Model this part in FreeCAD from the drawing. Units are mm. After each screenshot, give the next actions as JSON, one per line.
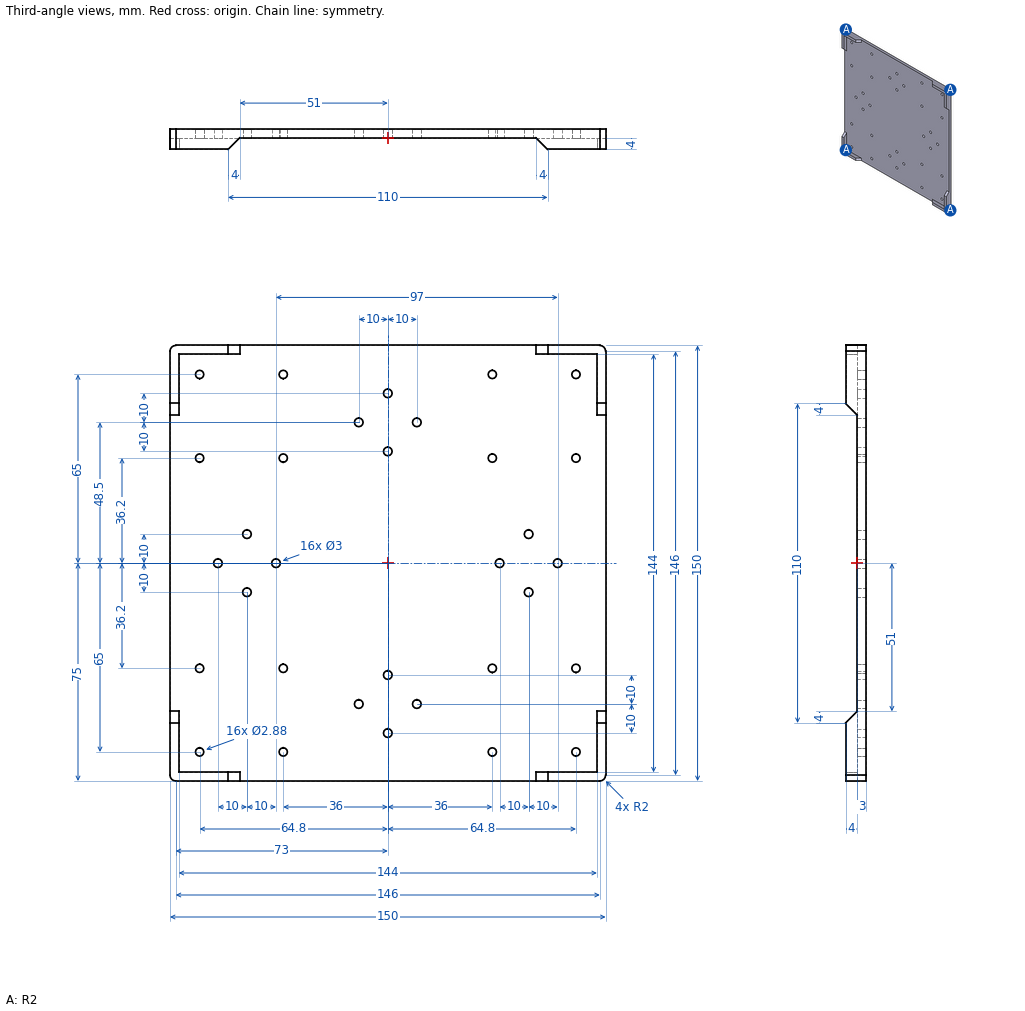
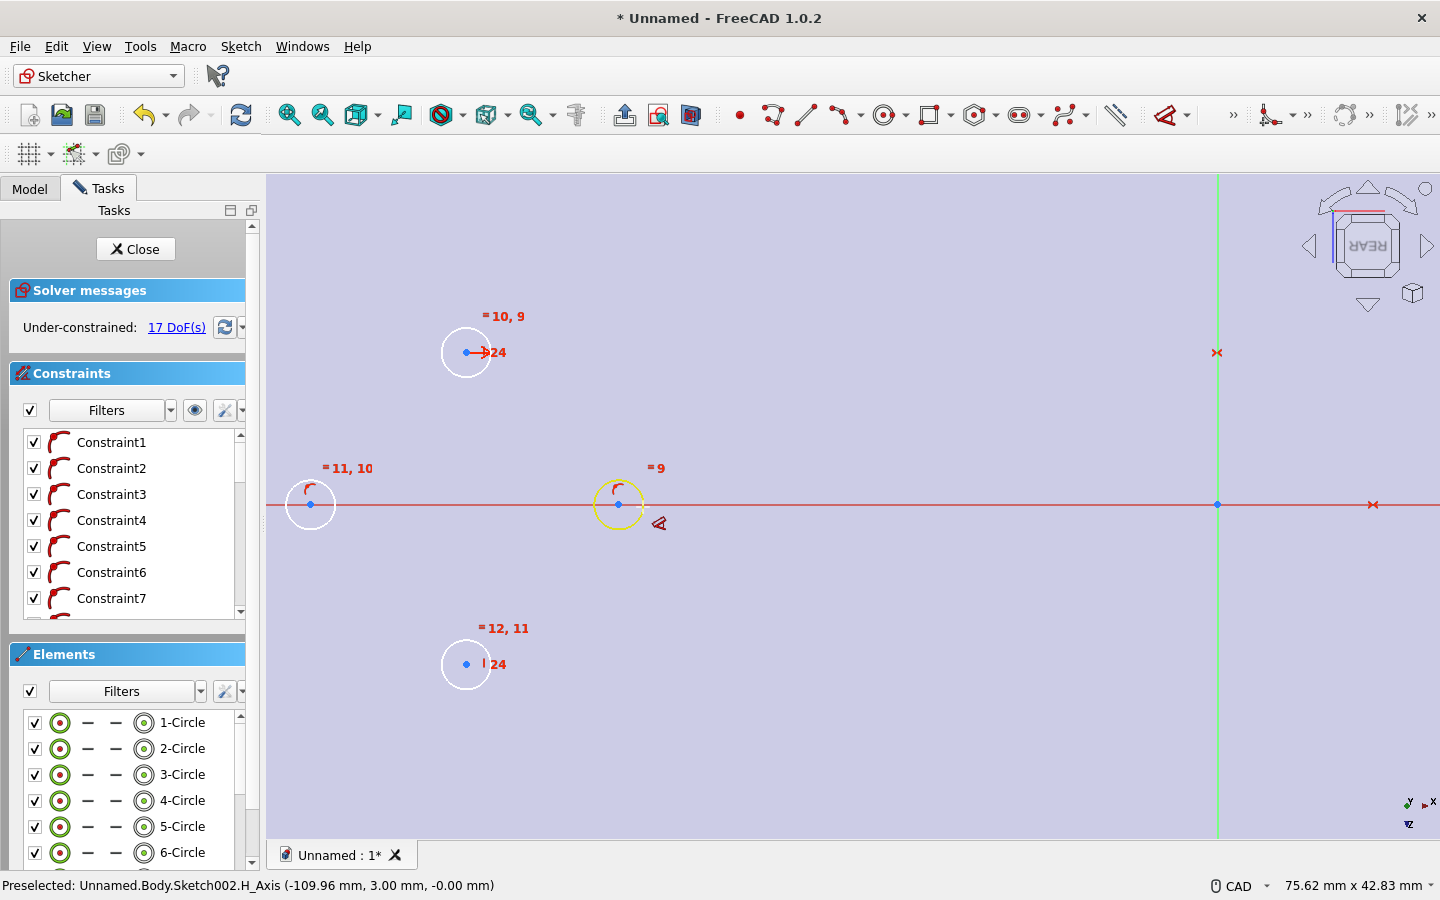
{"action": "left_click", "coordinate": [643, 506]}
{"action": "left_click", "coordinate": [667, 534]}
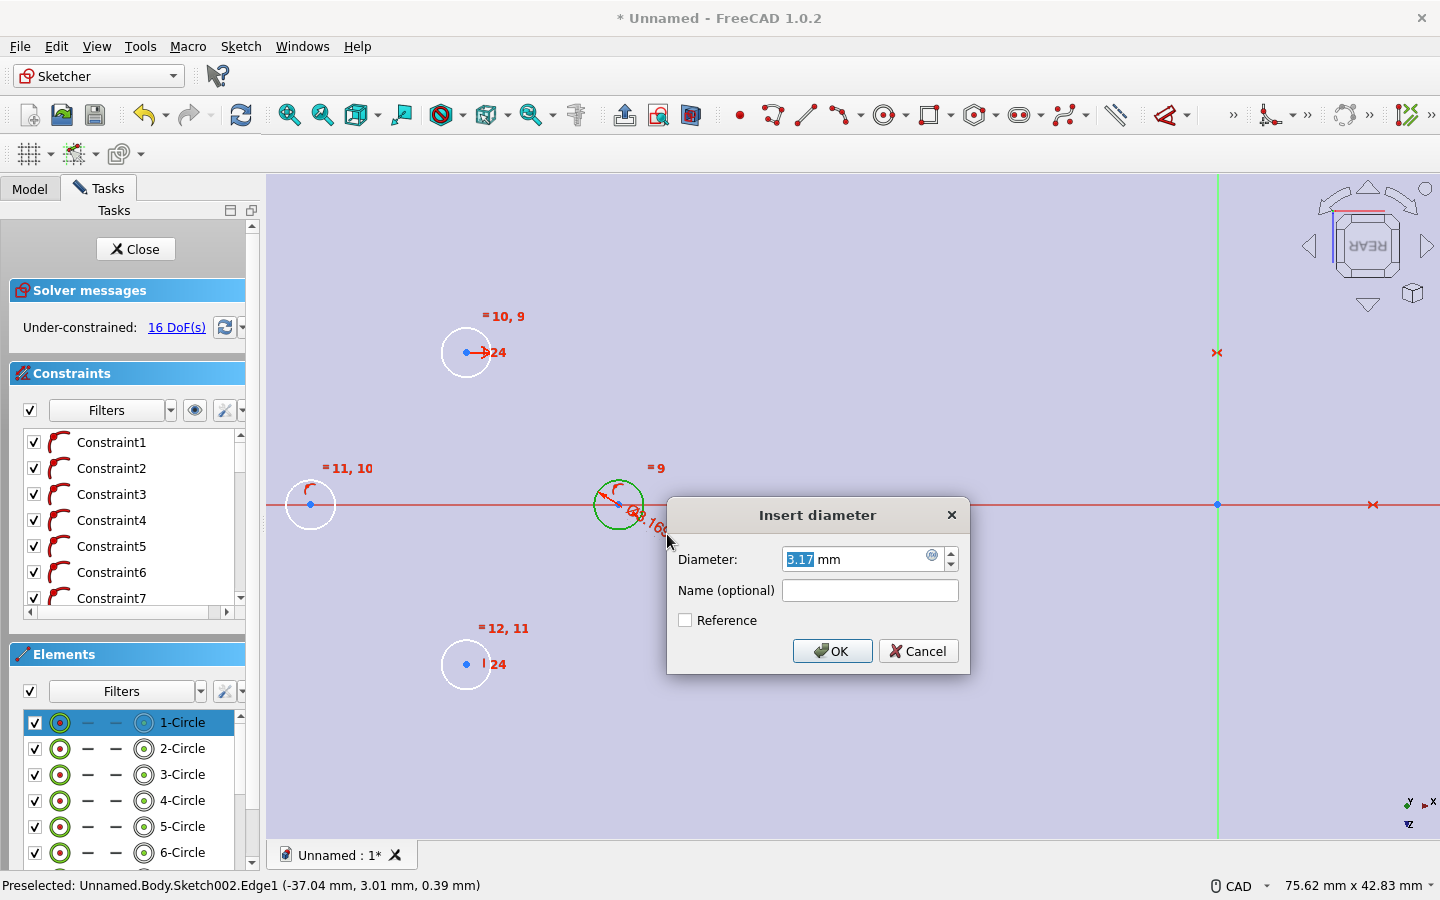
{"action": "type", "text": "3"}
{"action": "key", "text": "Return"}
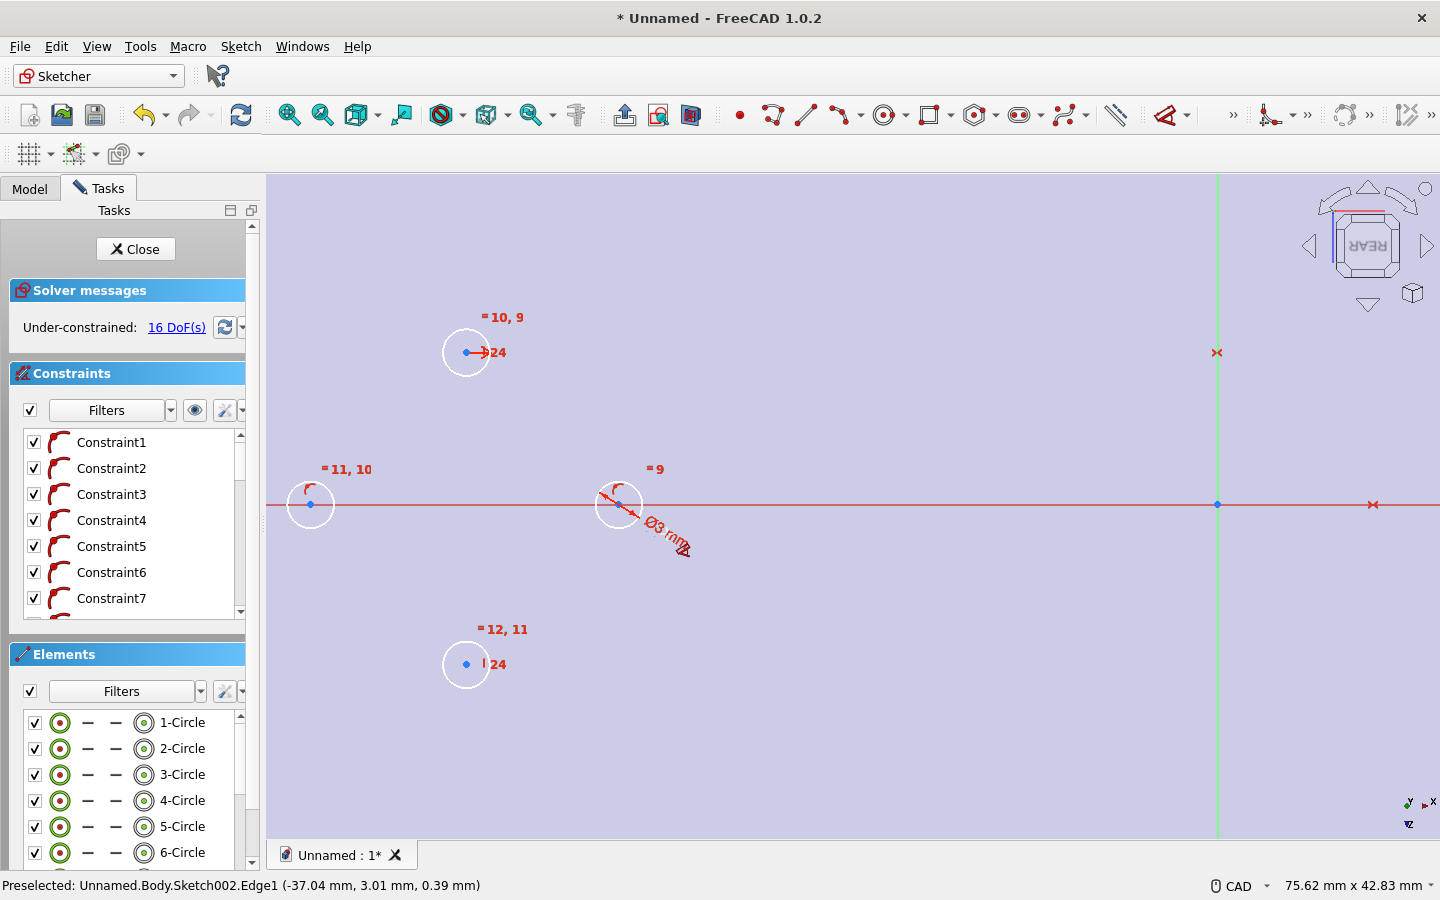
{"action": "scroll", "coordinate": [643, 507], "scroll_direction": "down", "scroll_amount": 7}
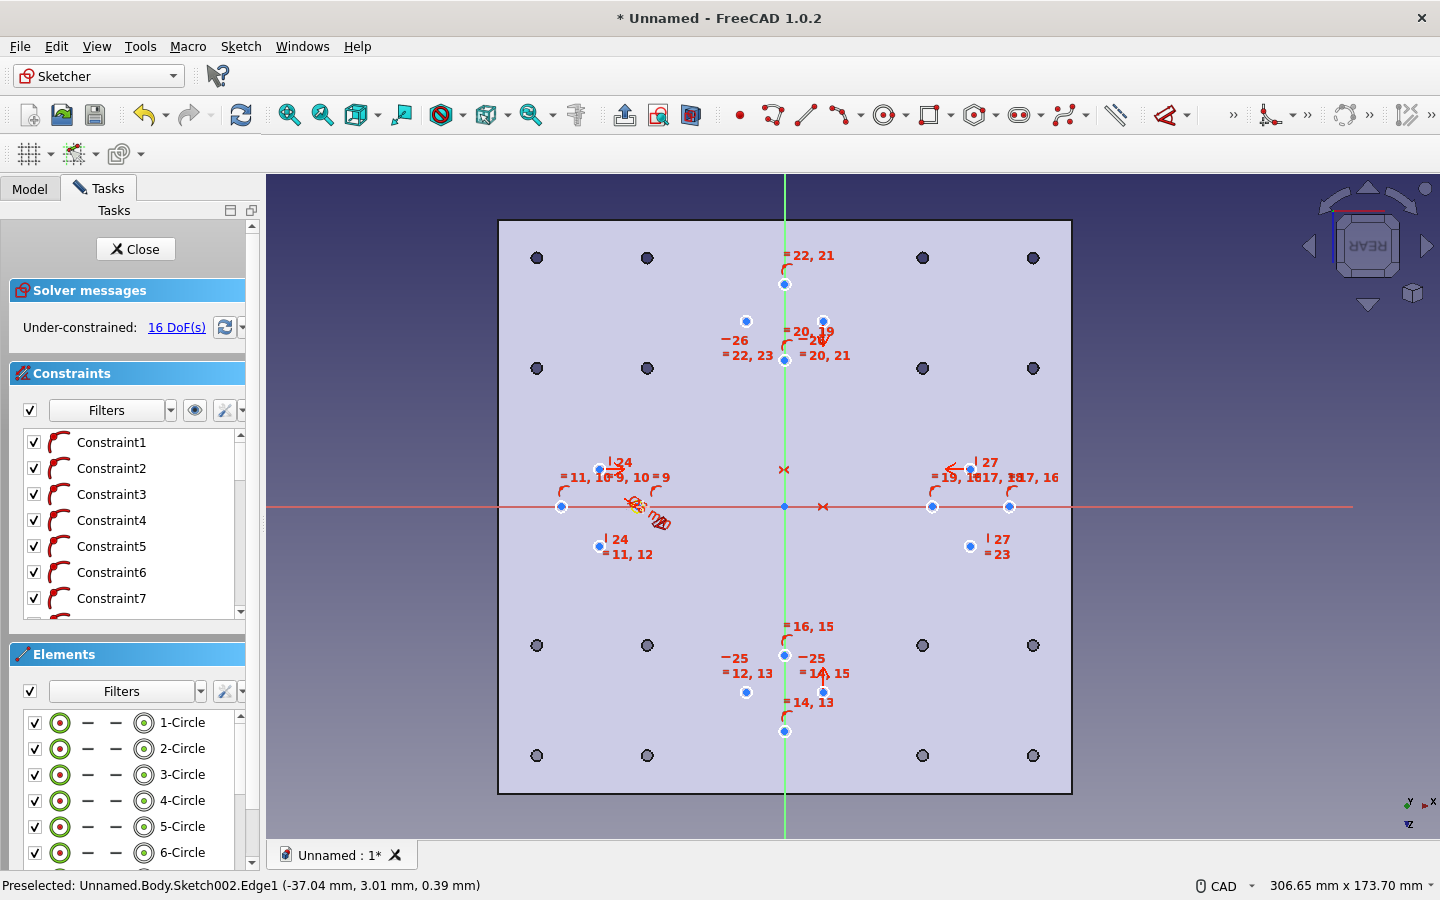
{"action": "left_click", "coordinate": [600, 469]}
{"action": "left_click", "coordinate": [566, 488]}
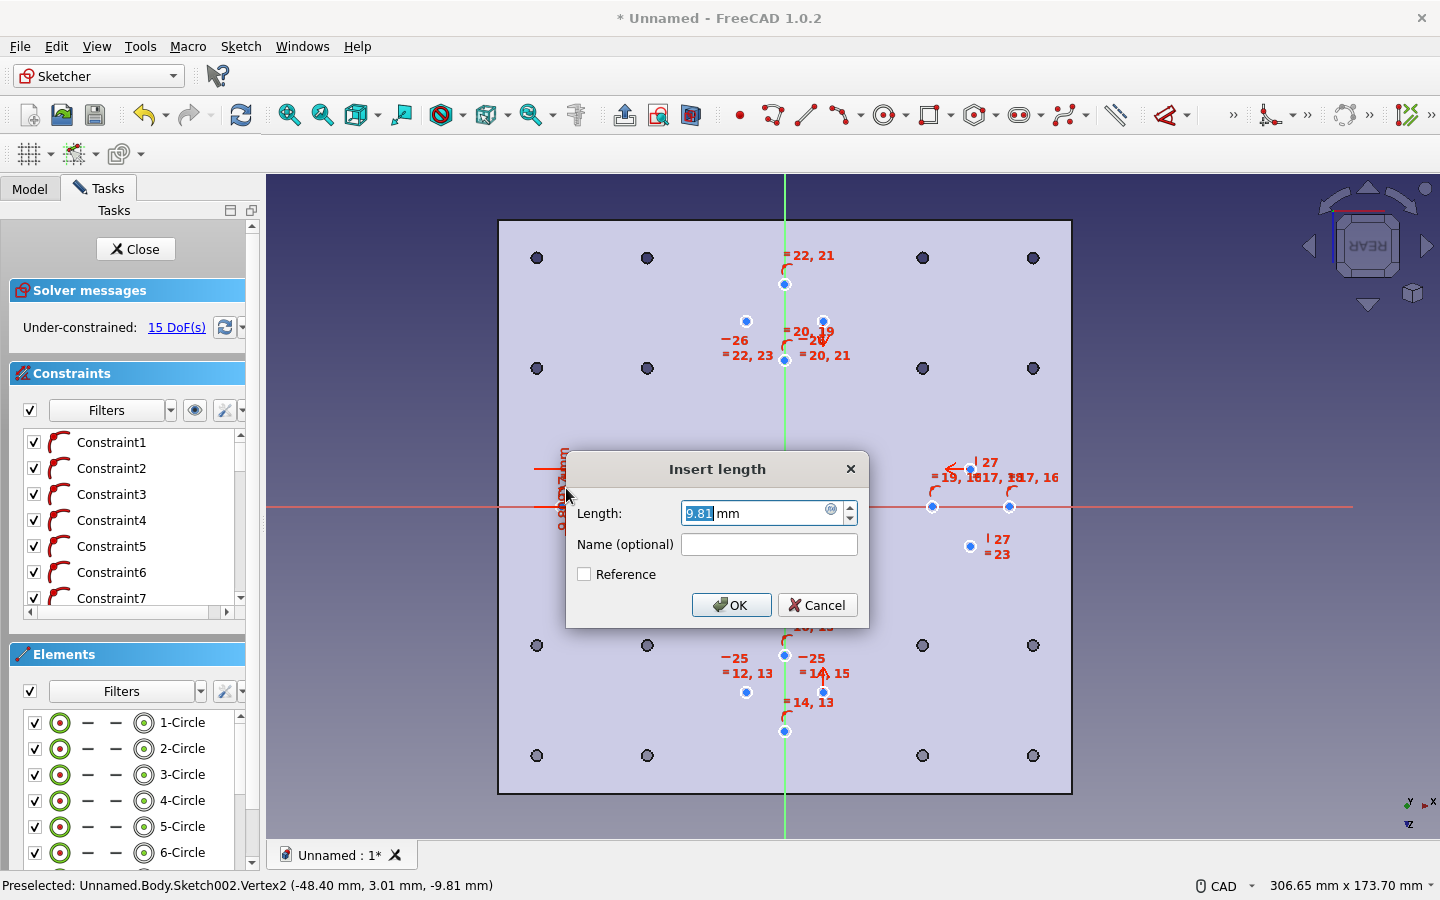
{"action": "type", "text": "10"}
{"action": "key", "text": "Return"}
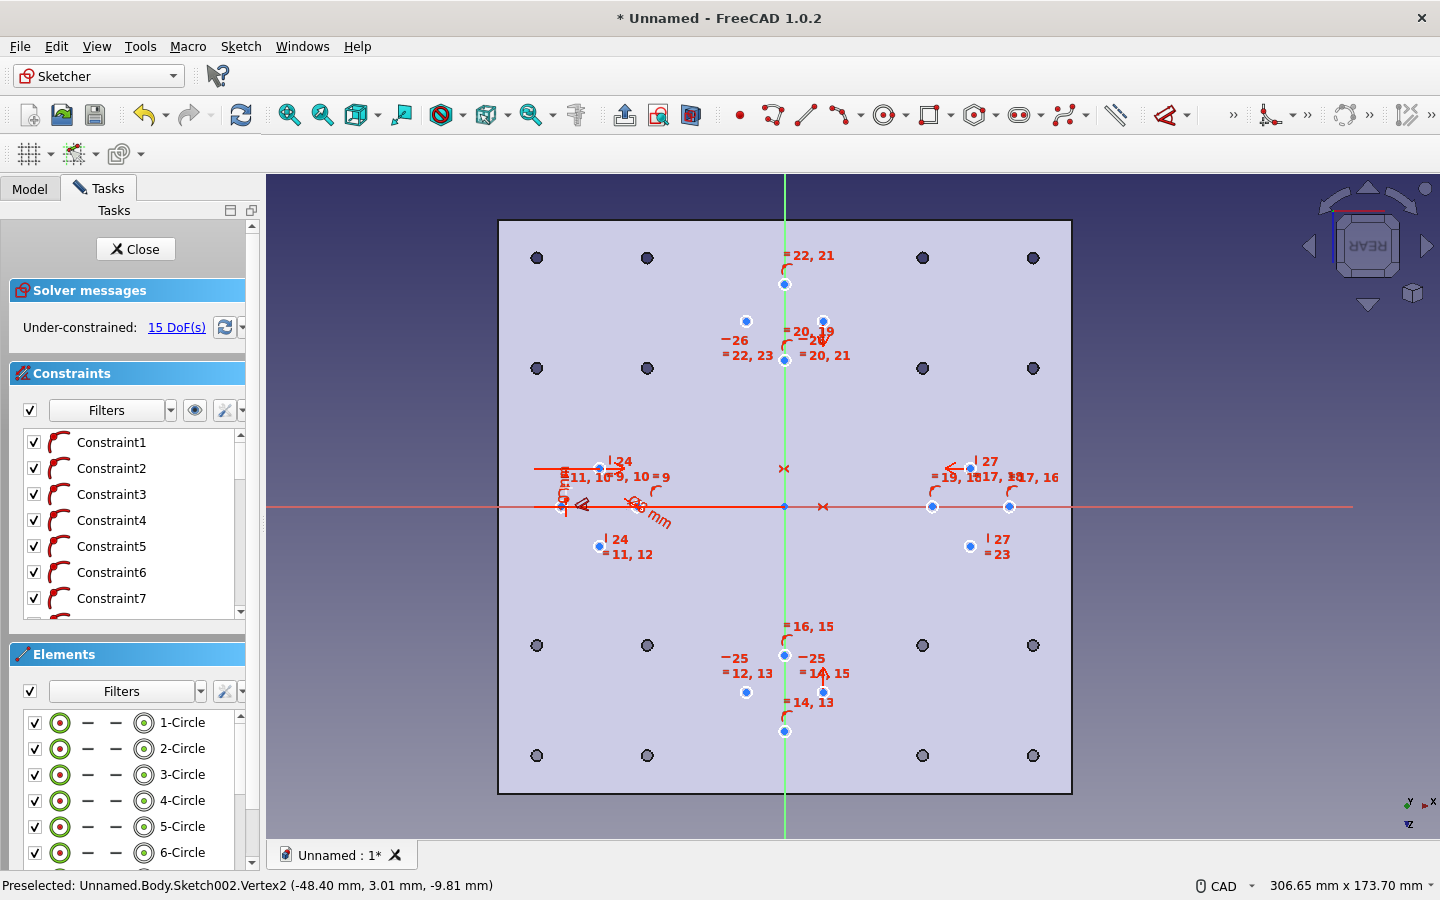
{"action": "left_click", "coordinate": [600, 546]}
{"action": "left_click", "coordinate": [566, 527]}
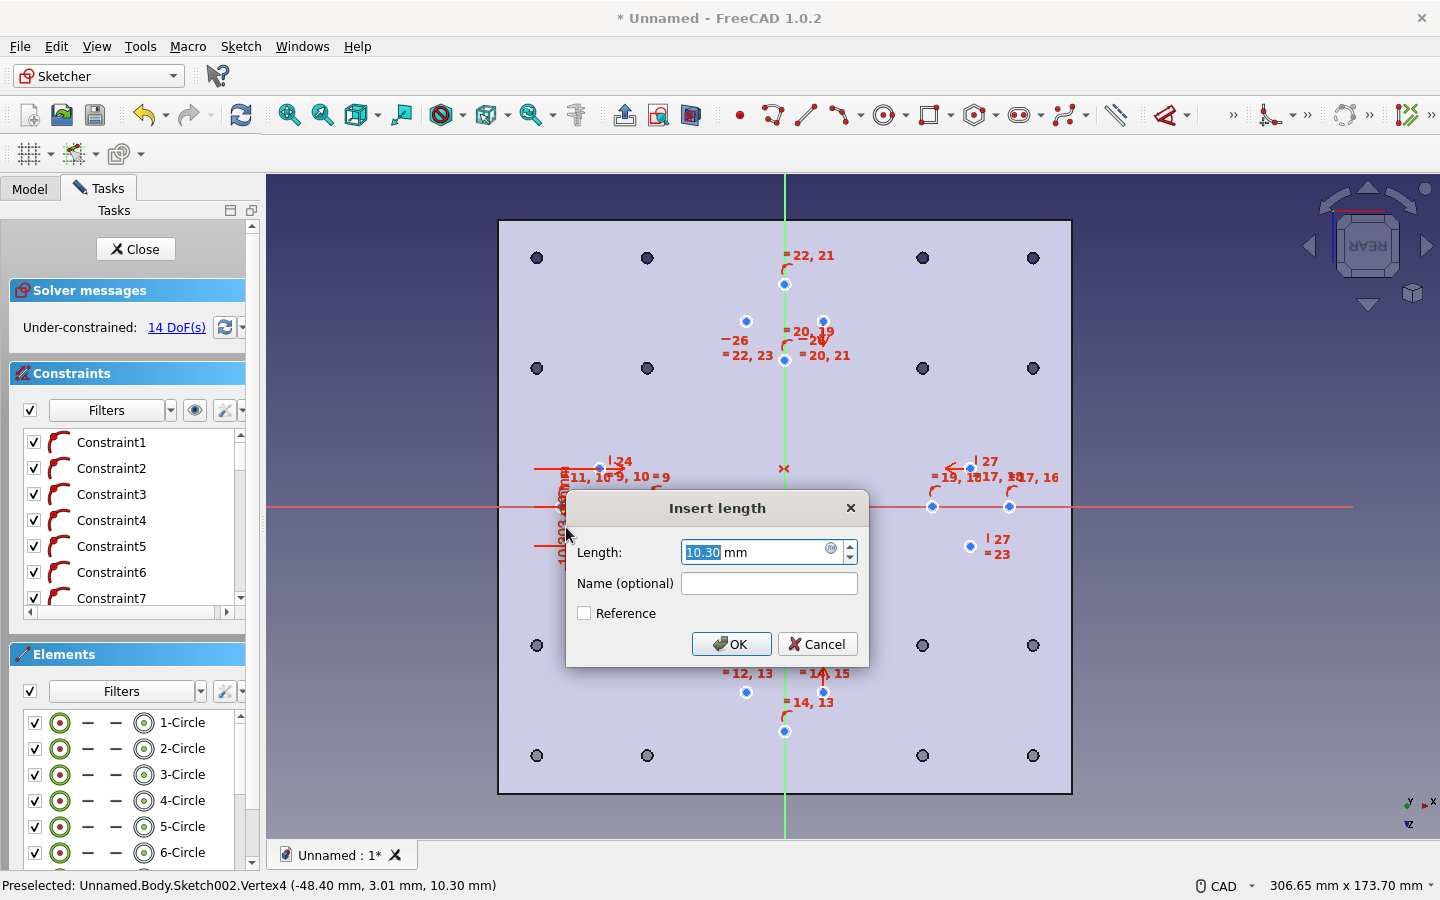
{"action": "type", "text": "10"}
{"action": "key", "text": "Return"}